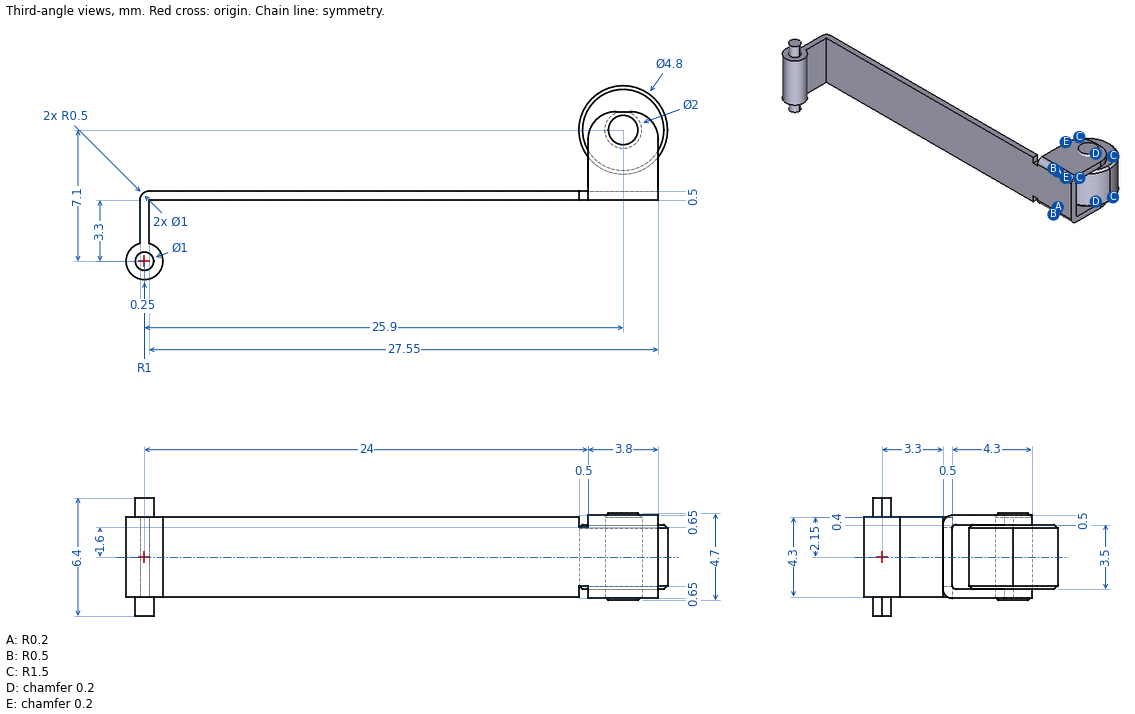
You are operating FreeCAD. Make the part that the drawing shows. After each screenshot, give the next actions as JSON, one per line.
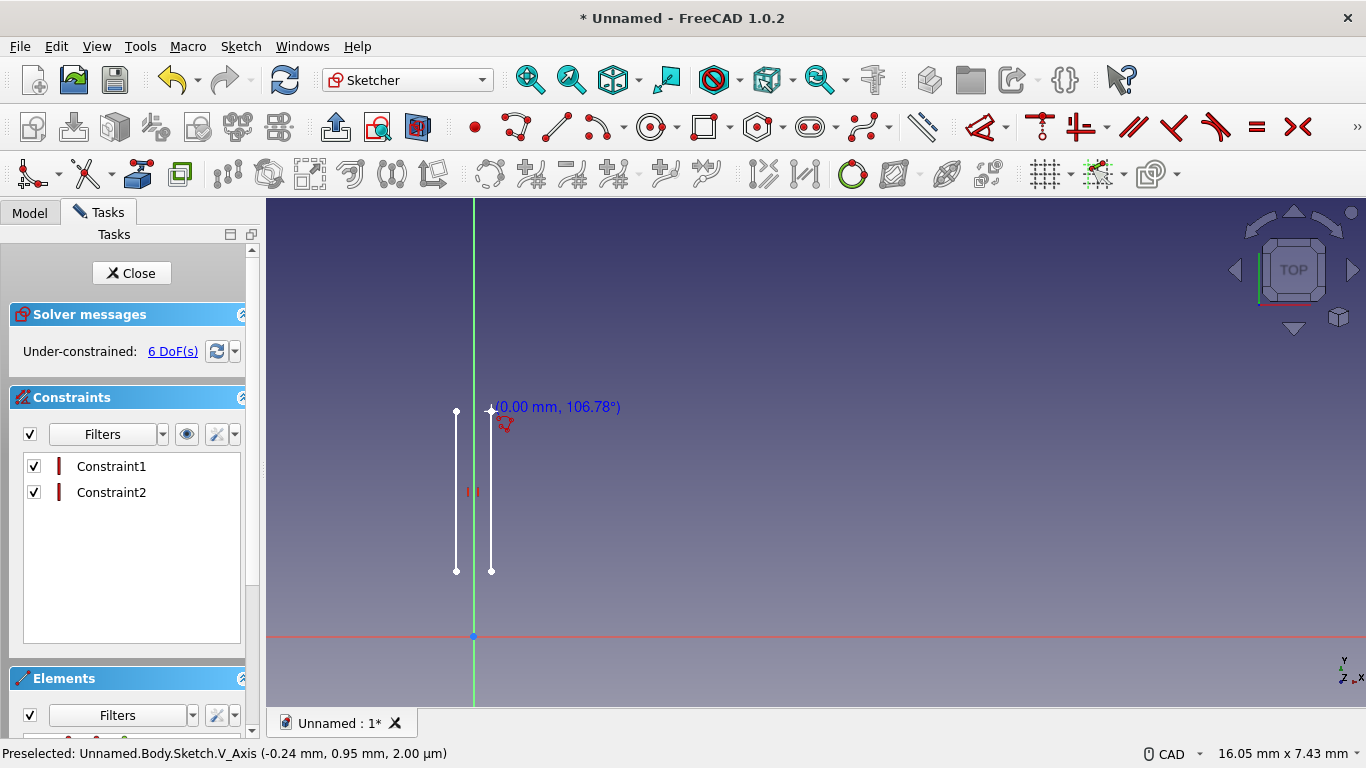
{"action": "scroll", "coordinate": [462, 414], "scroll_direction": "down", "scroll_amount": 6}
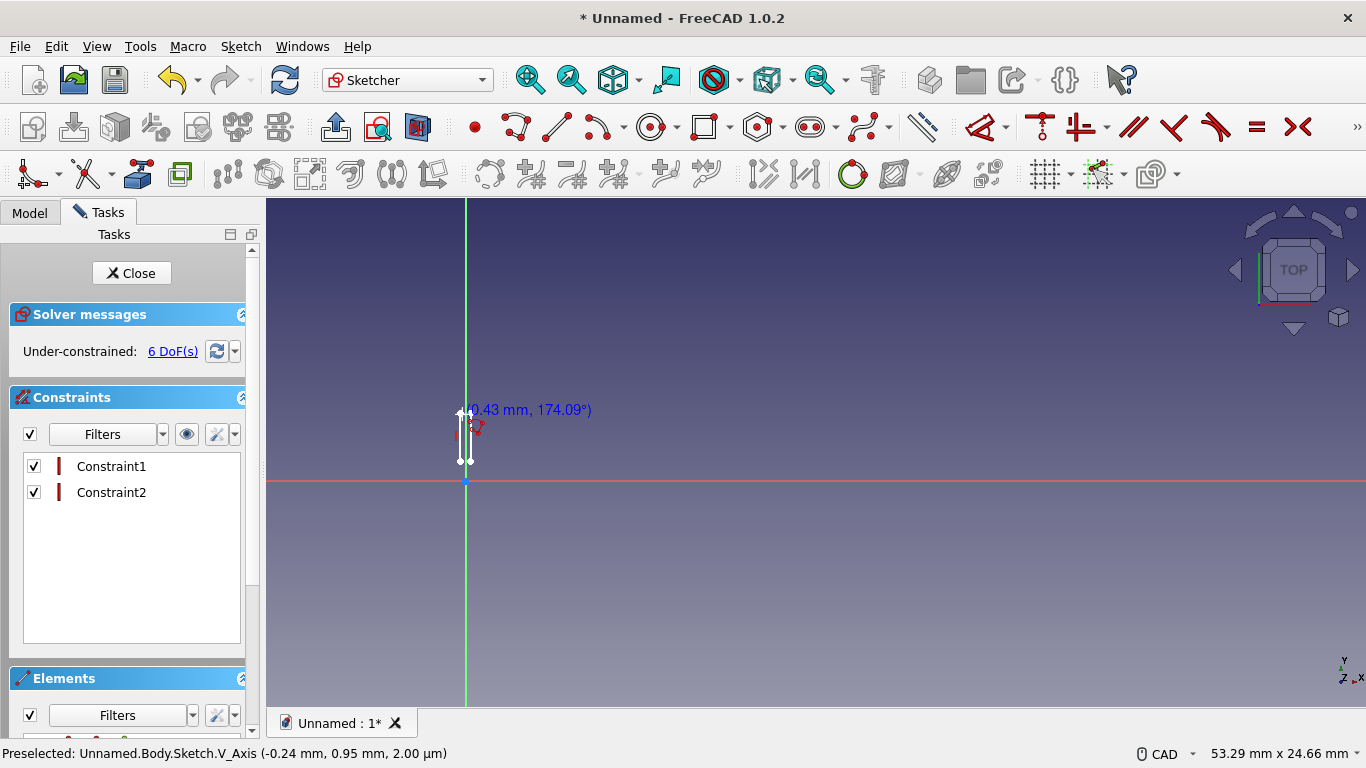
{"action": "left_click", "coordinate": [1039, 413]}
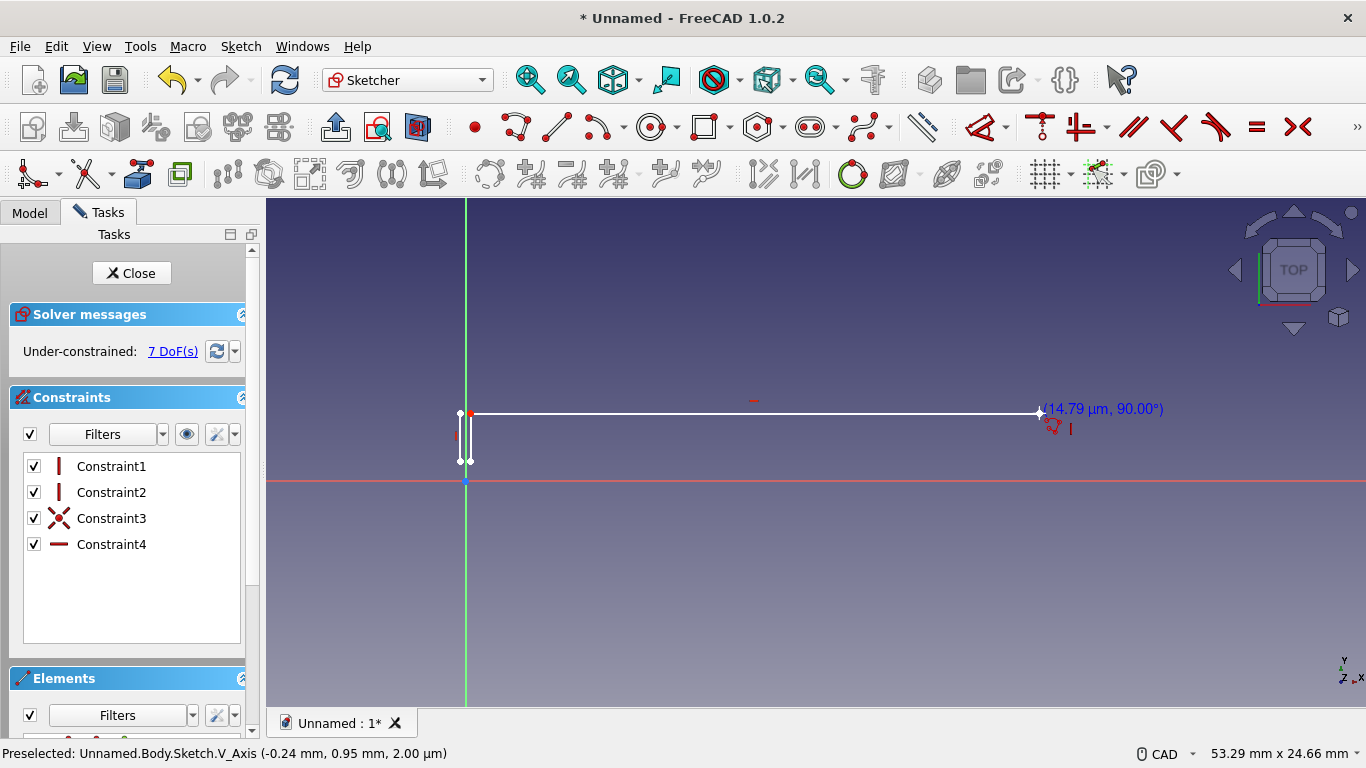
{"action": "scroll", "coordinate": [1039, 403], "scroll_direction": "up", "scroll_amount": 3}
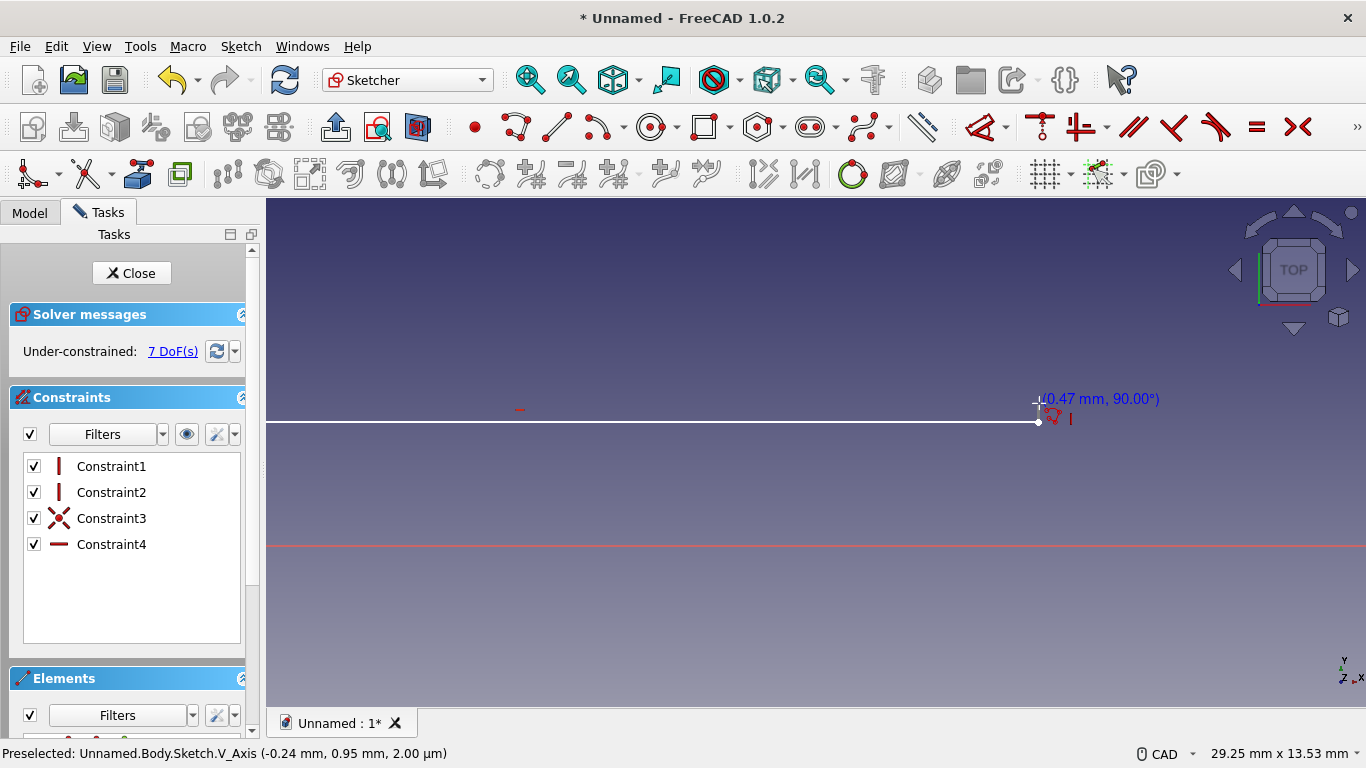
{"action": "left_click", "coordinate": [1038, 403]}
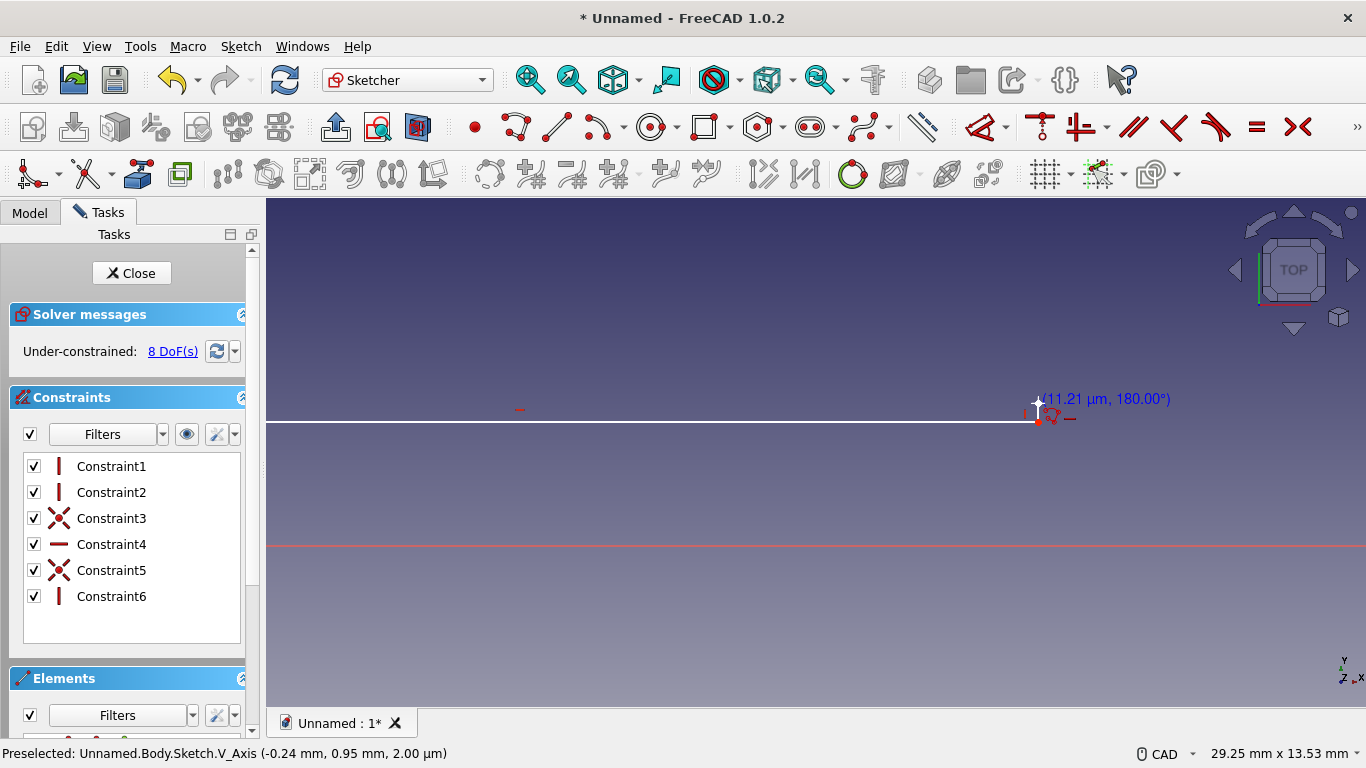
{"action": "scroll", "coordinate": [1040, 403], "scroll_direction": "down", "scroll_amount": 3}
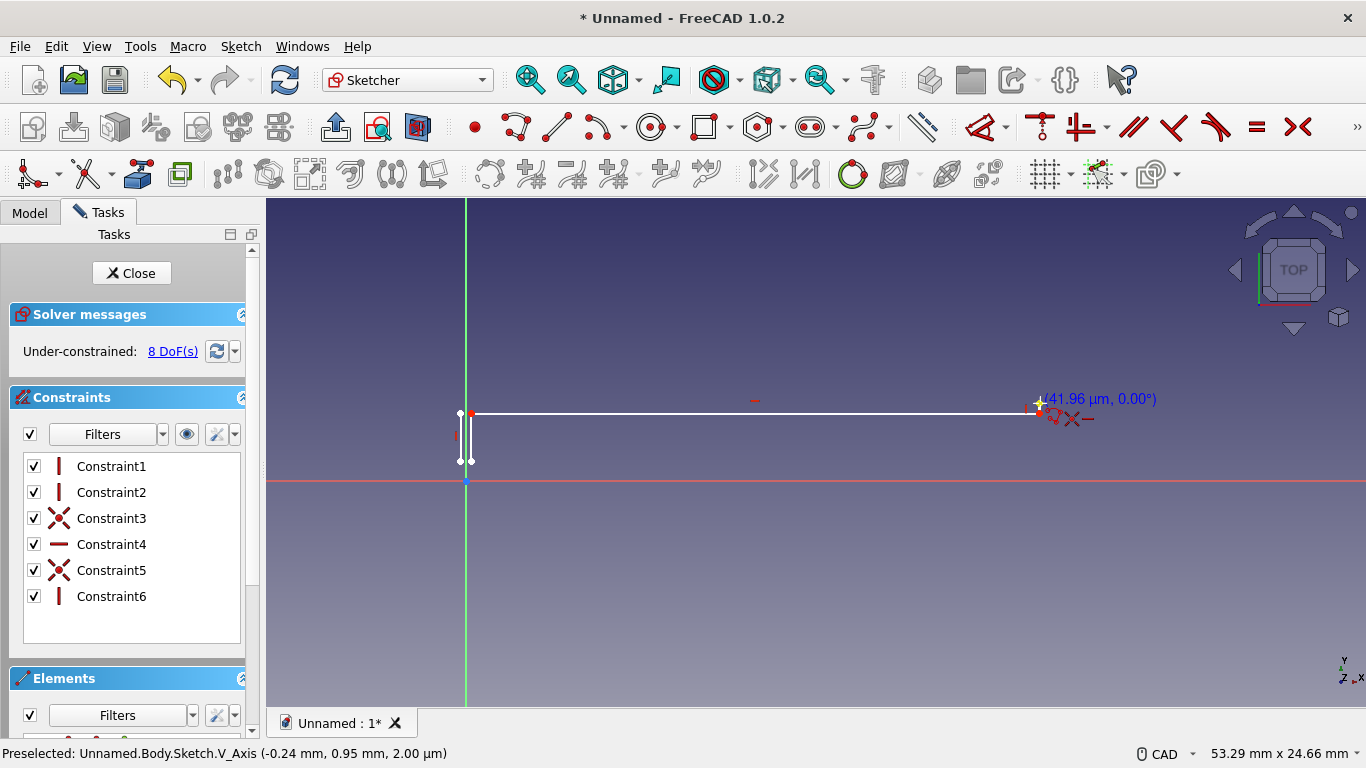
{"action": "scroll", "coordinate": [471, 403], "scroll_direction": "up", "scroll_amount": 6}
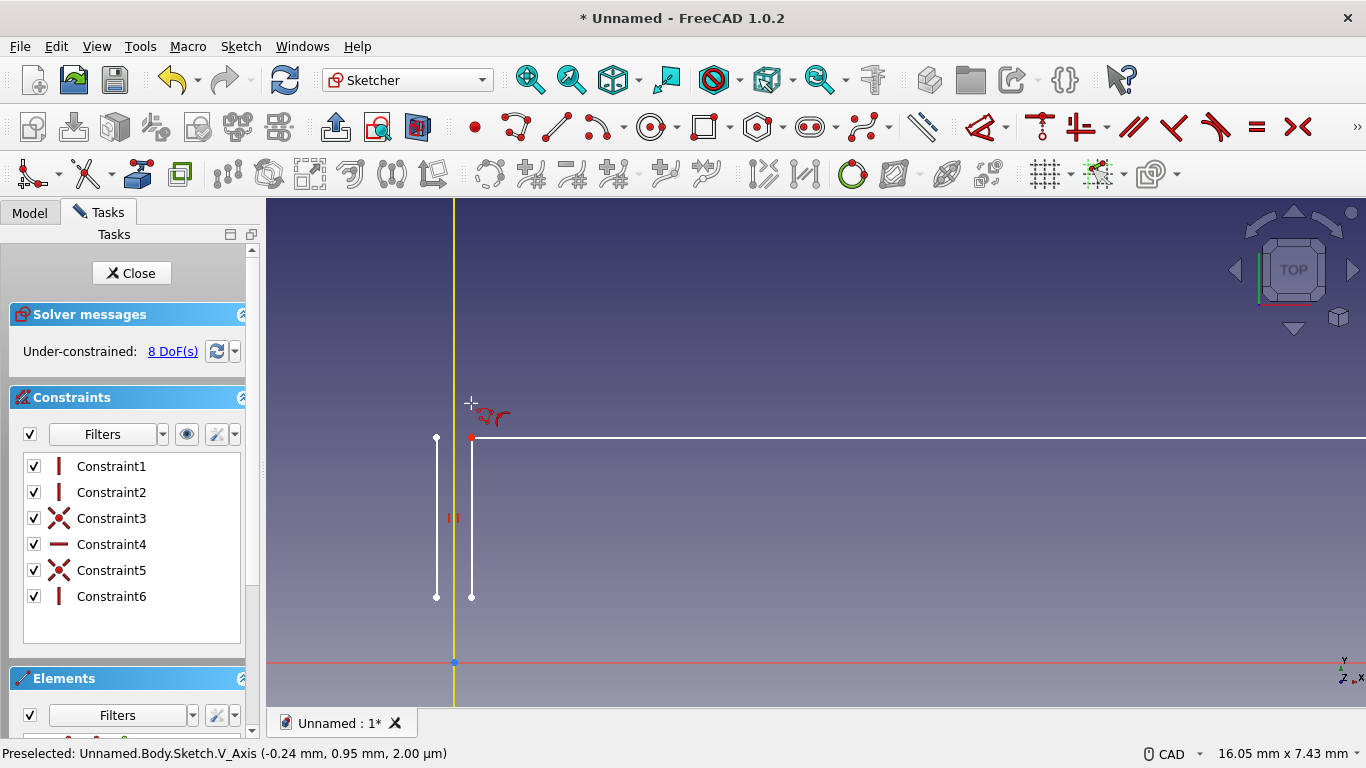
{"action": "left_click", "coordinate": [471, 403]}
{"action": "right_click", "coordinate": [471, 403]}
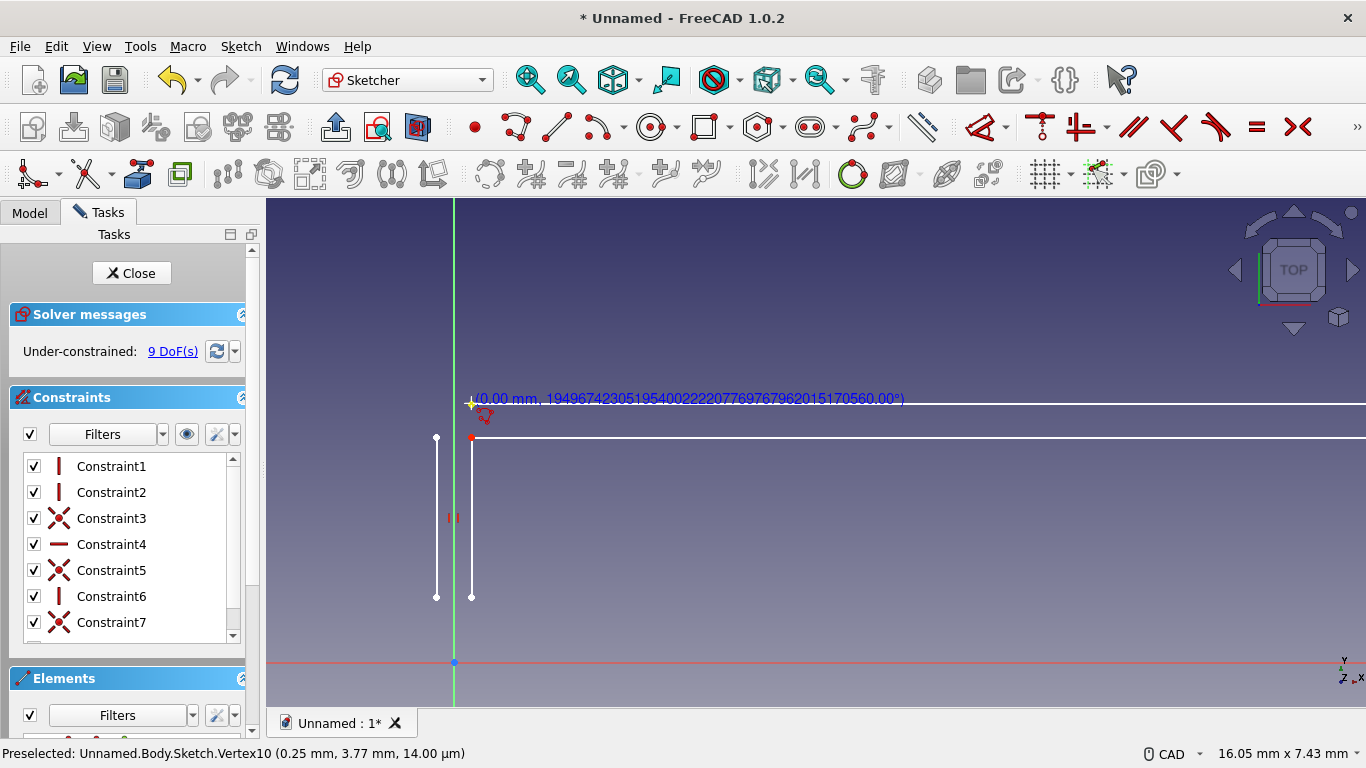
{"action": "key", "text": "g 3 a"}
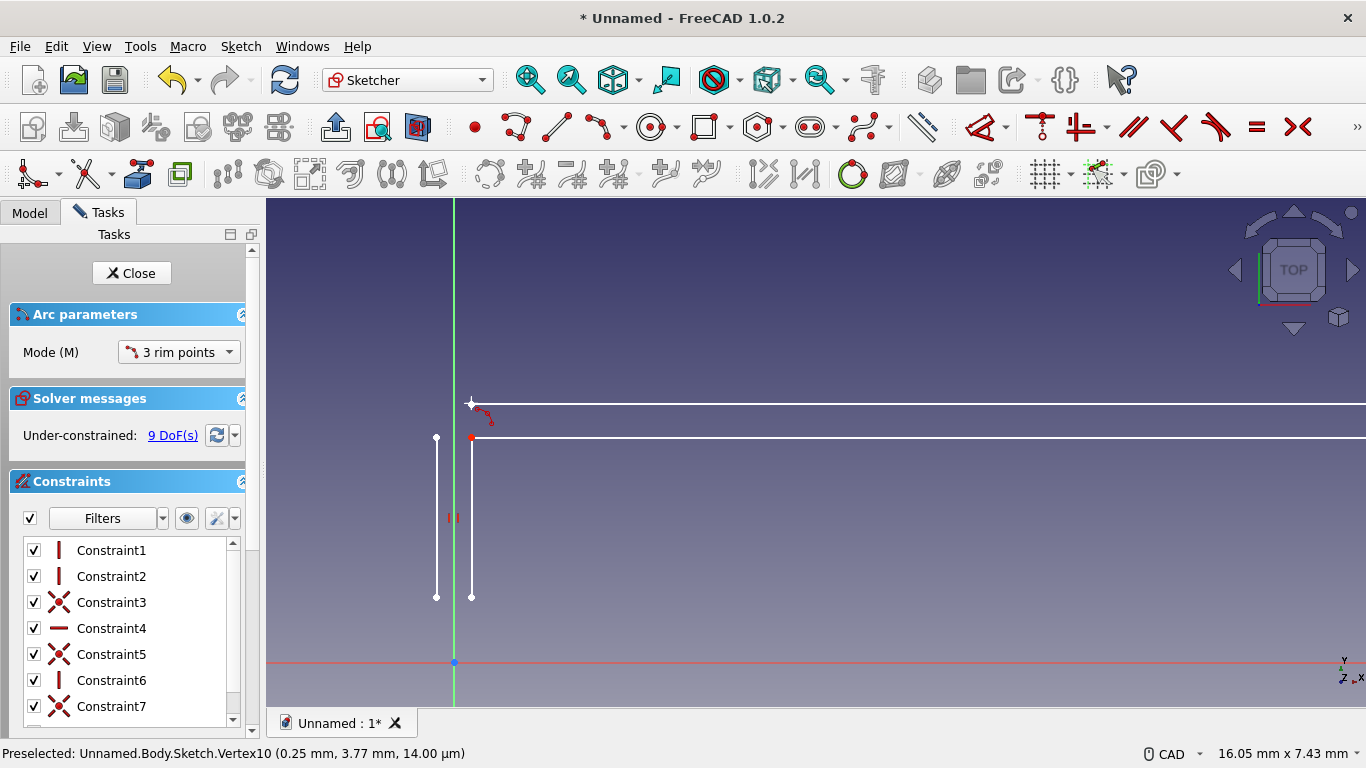
{"action": "left_click", "coordinate": [437, 598]}
{"action": "left_click", "coordinate": [472, 598]}